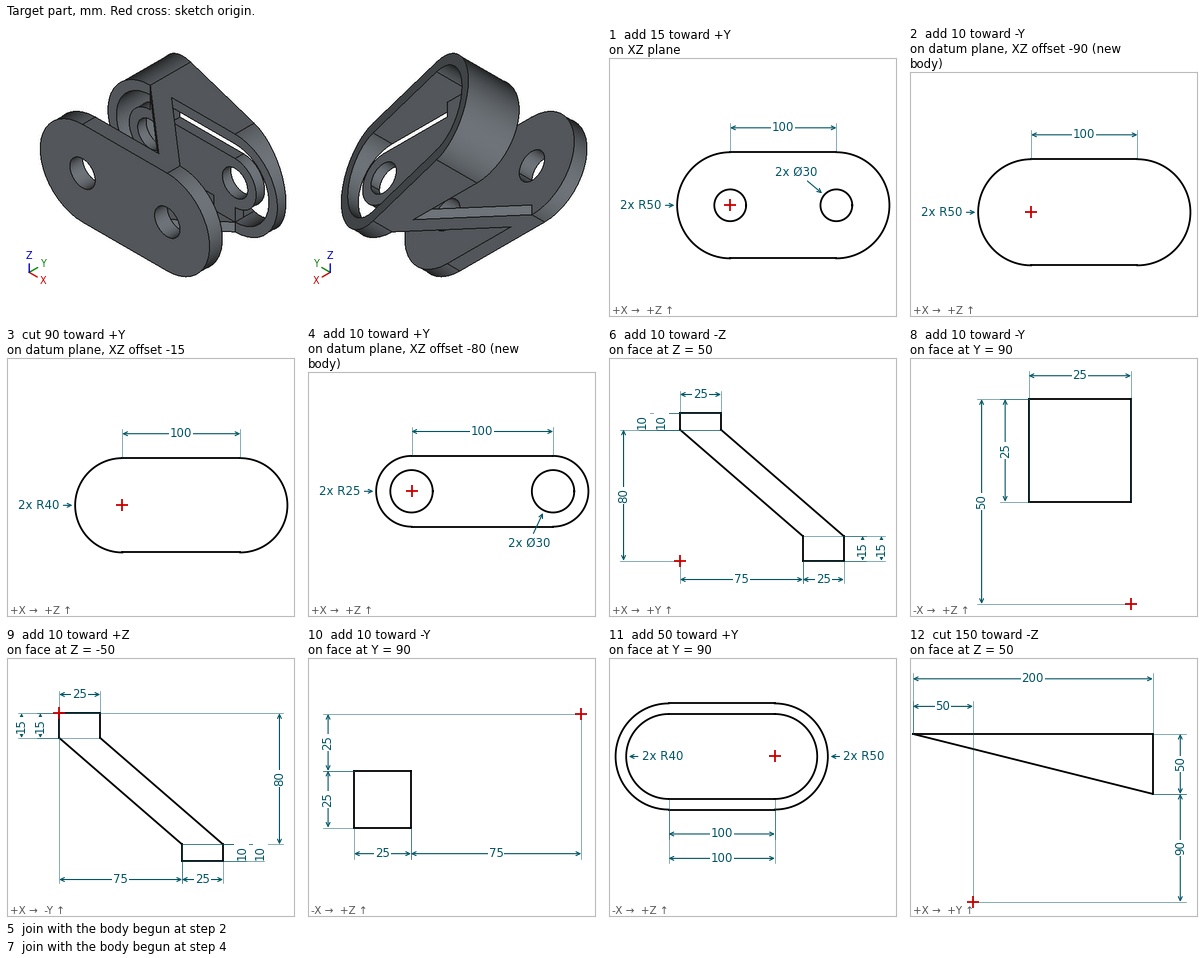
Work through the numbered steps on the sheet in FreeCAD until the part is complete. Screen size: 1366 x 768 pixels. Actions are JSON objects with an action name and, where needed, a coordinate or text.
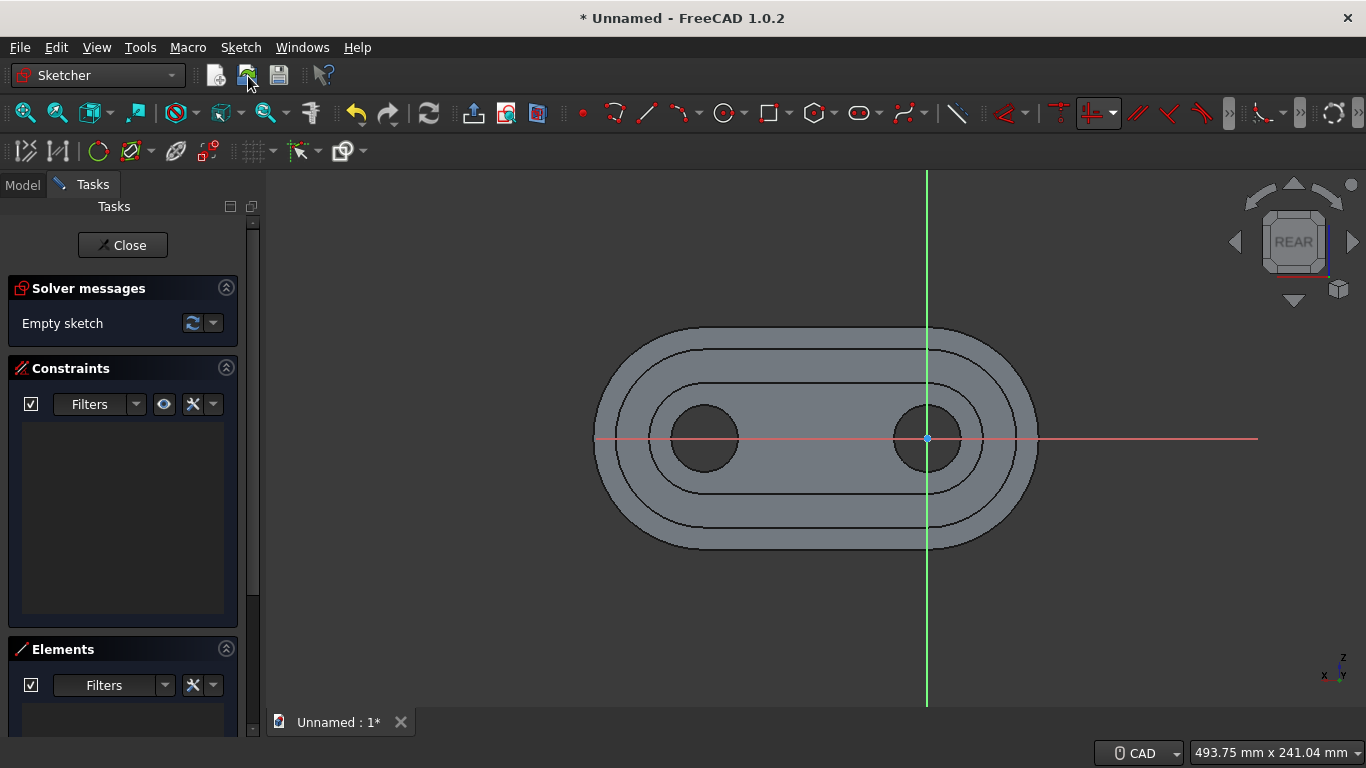
{"action": "scroll", "coordinate": [965, 359], "scroll_direction": "up", "scroll_amount": 6}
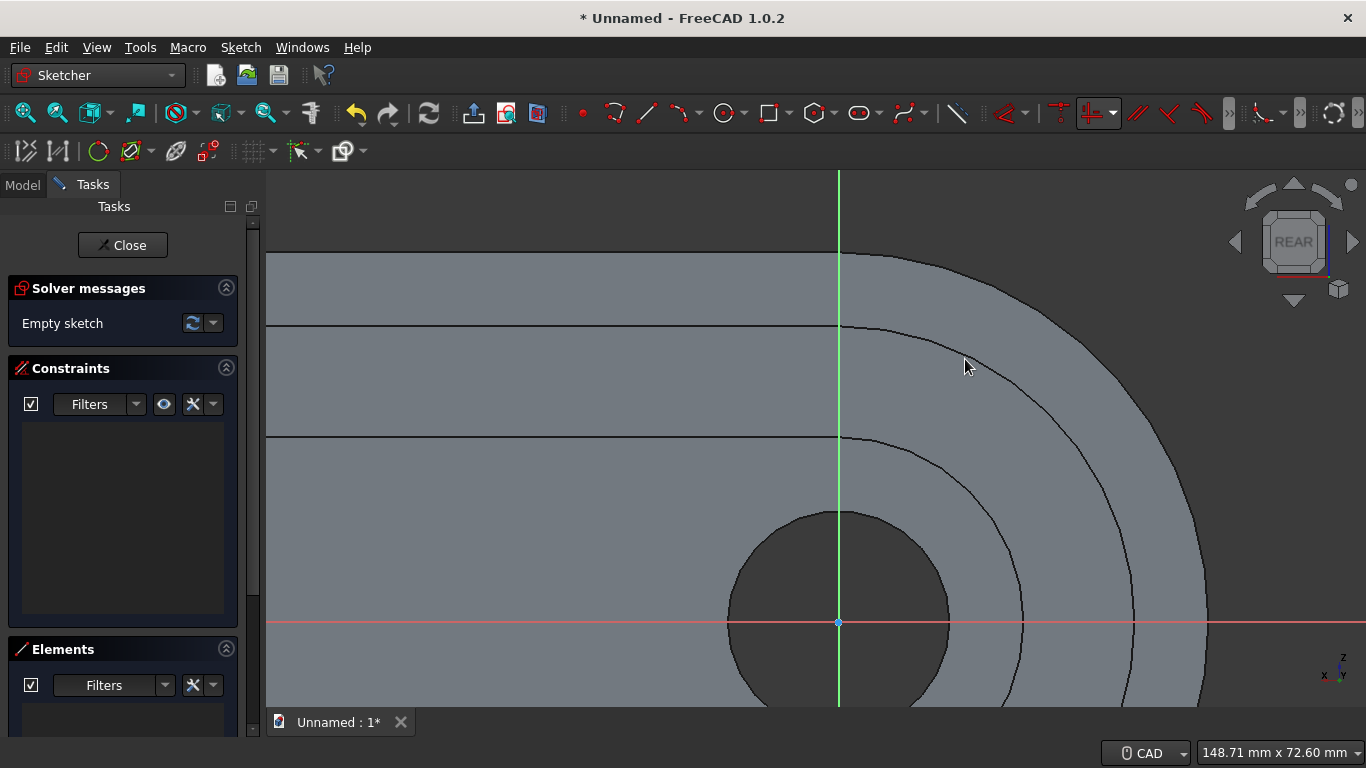
{"action": "left_click", "coordinate": [770, 114]}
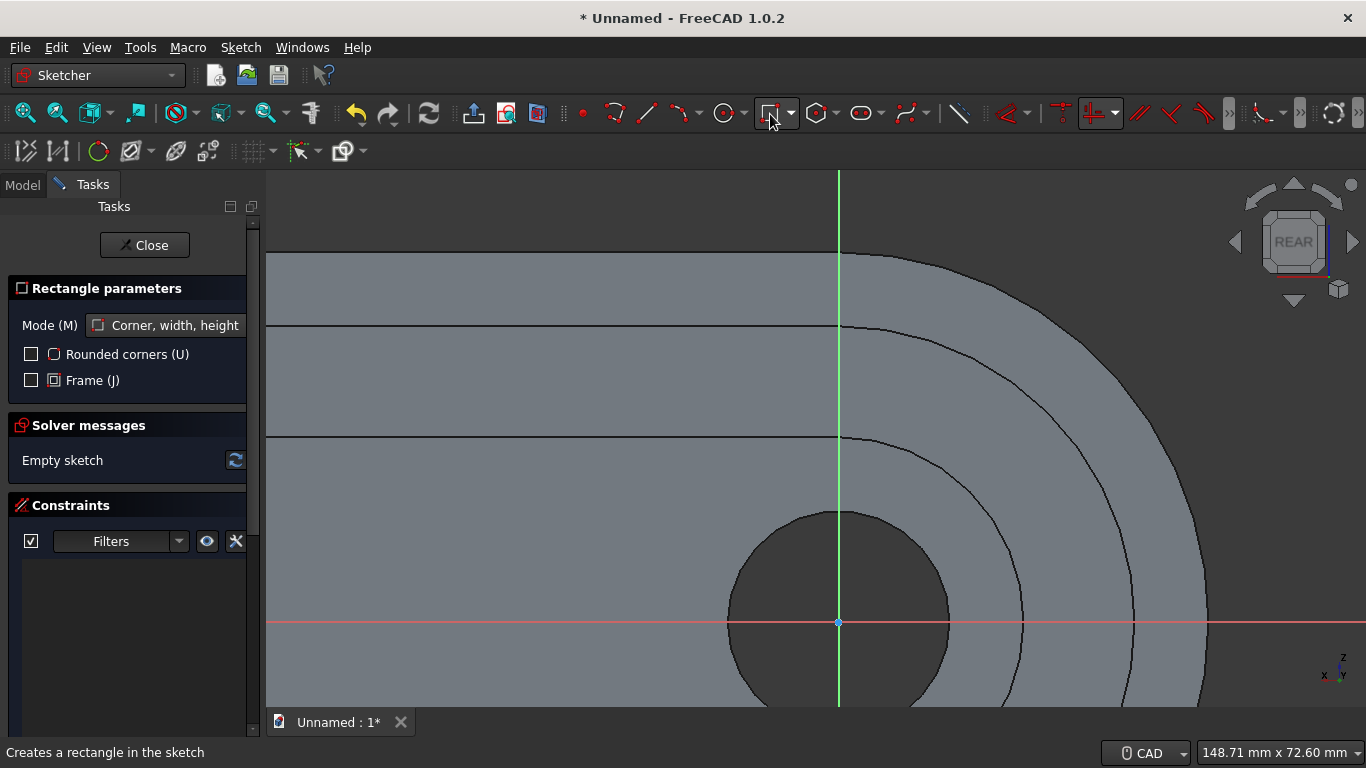
{"action": "left_click", "coordinate": [654, 252]}
{"action": "left_click", "coordinate": [839, 437]}
{"action": "key", "text": "Escape"}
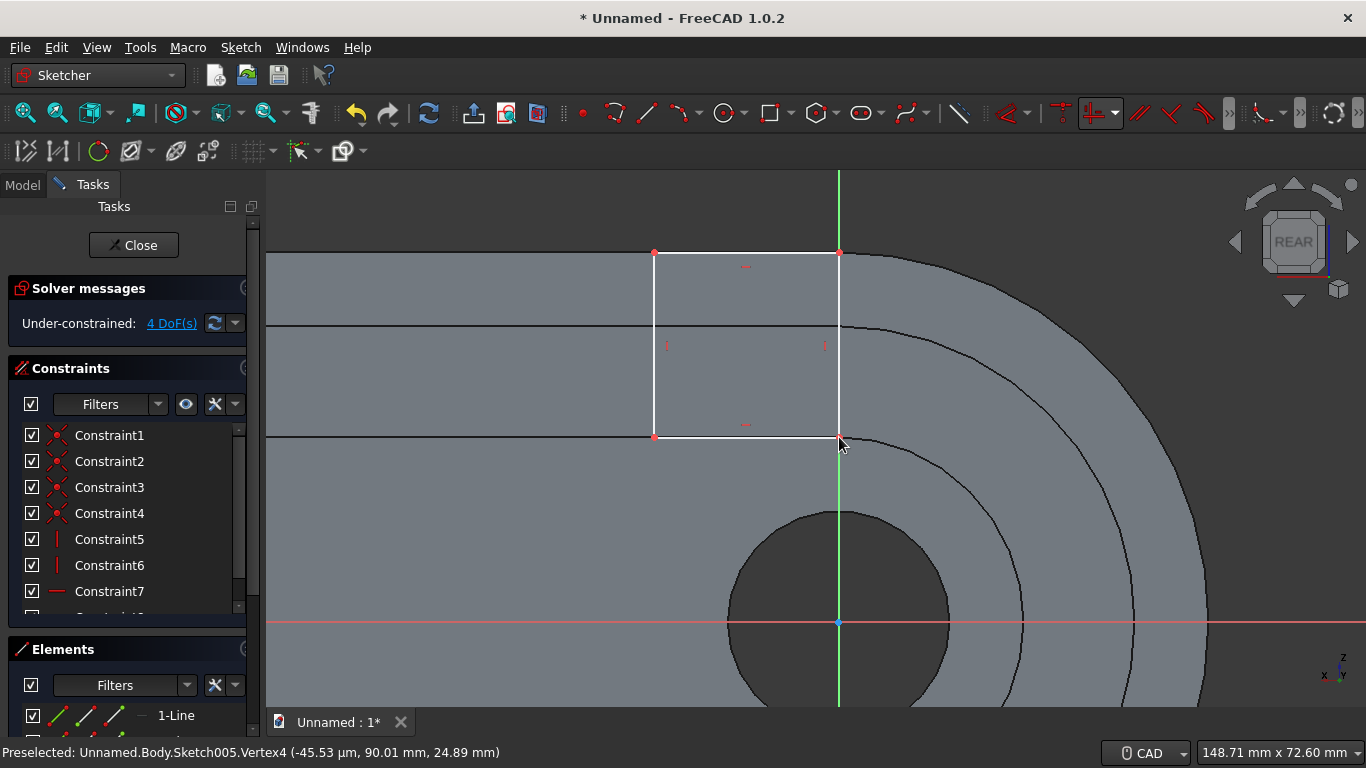
{"action": "left_click", "coordinate": [839, 438]}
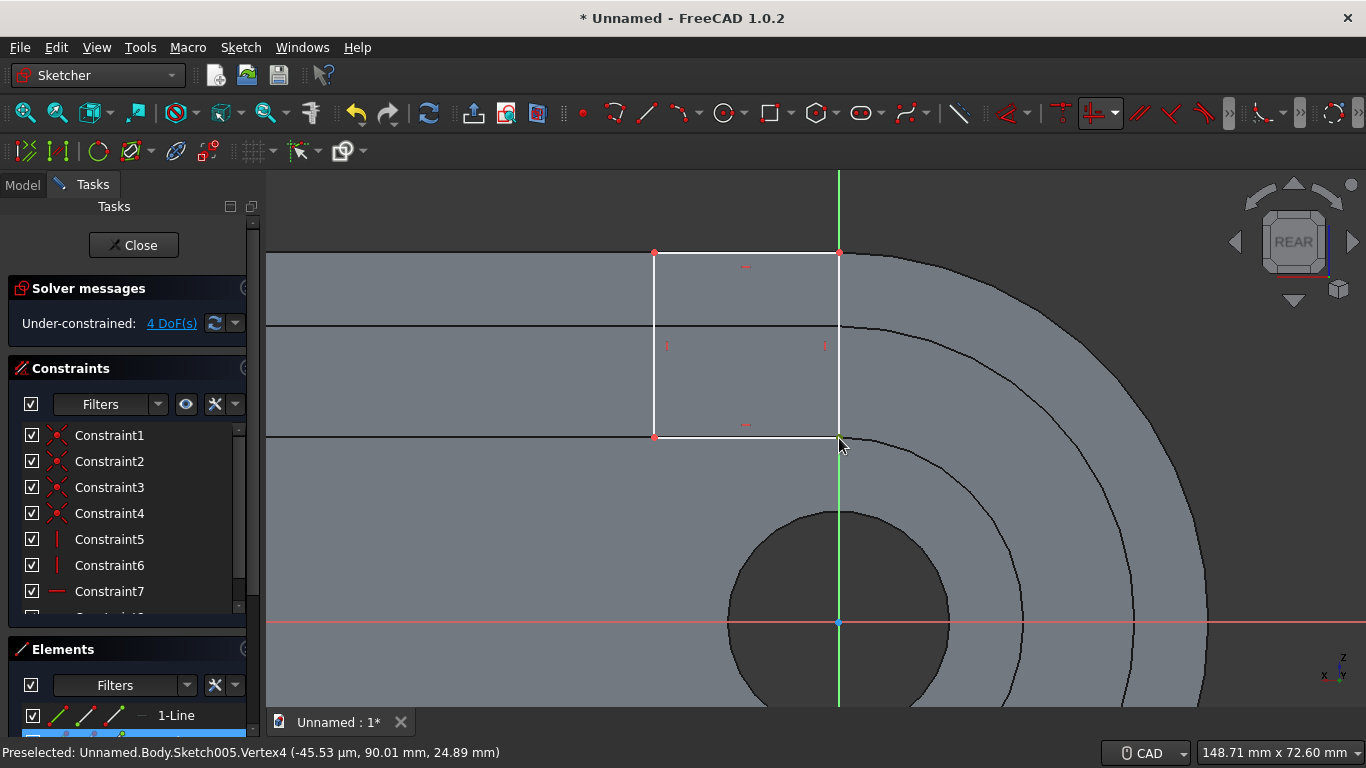
{"action": "left_click", "coordinate": [839, 576]}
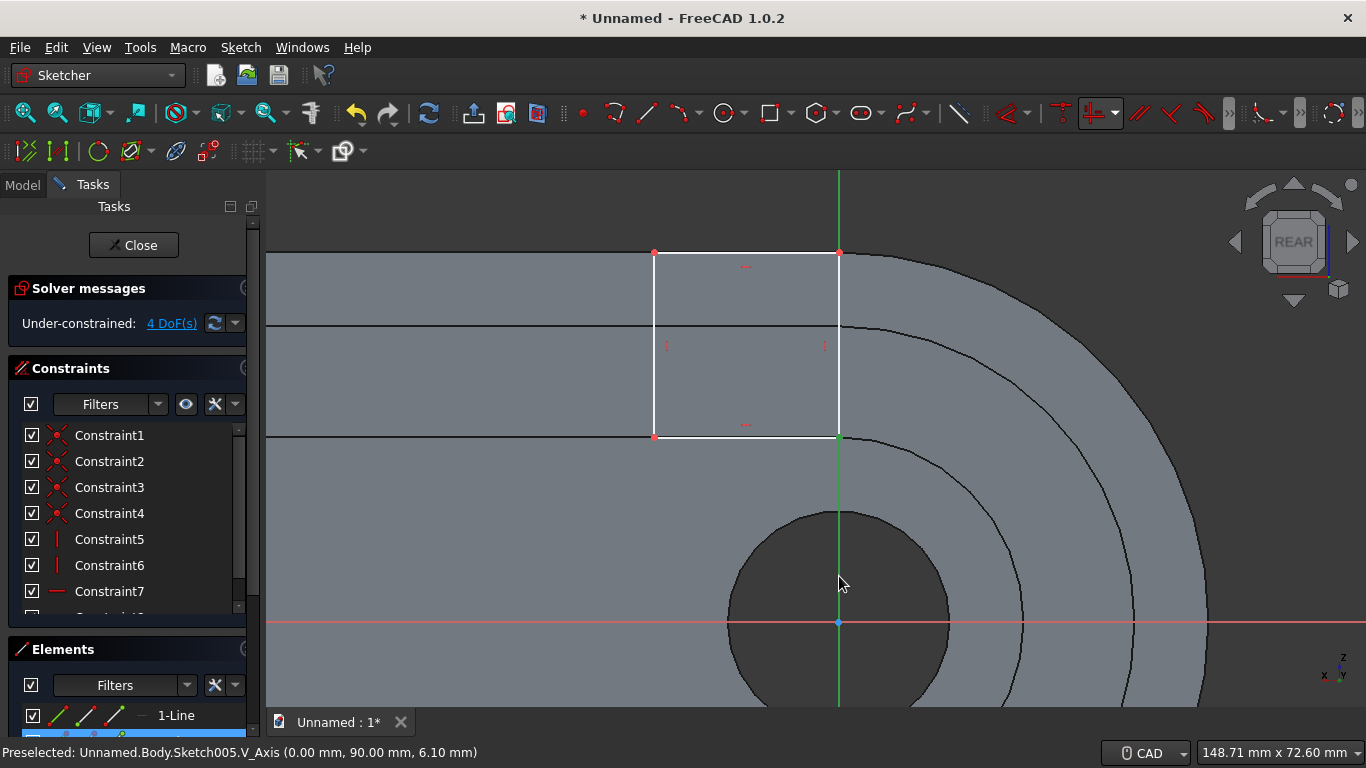
{"action": "left_click", "coordinate": [1062, 114]}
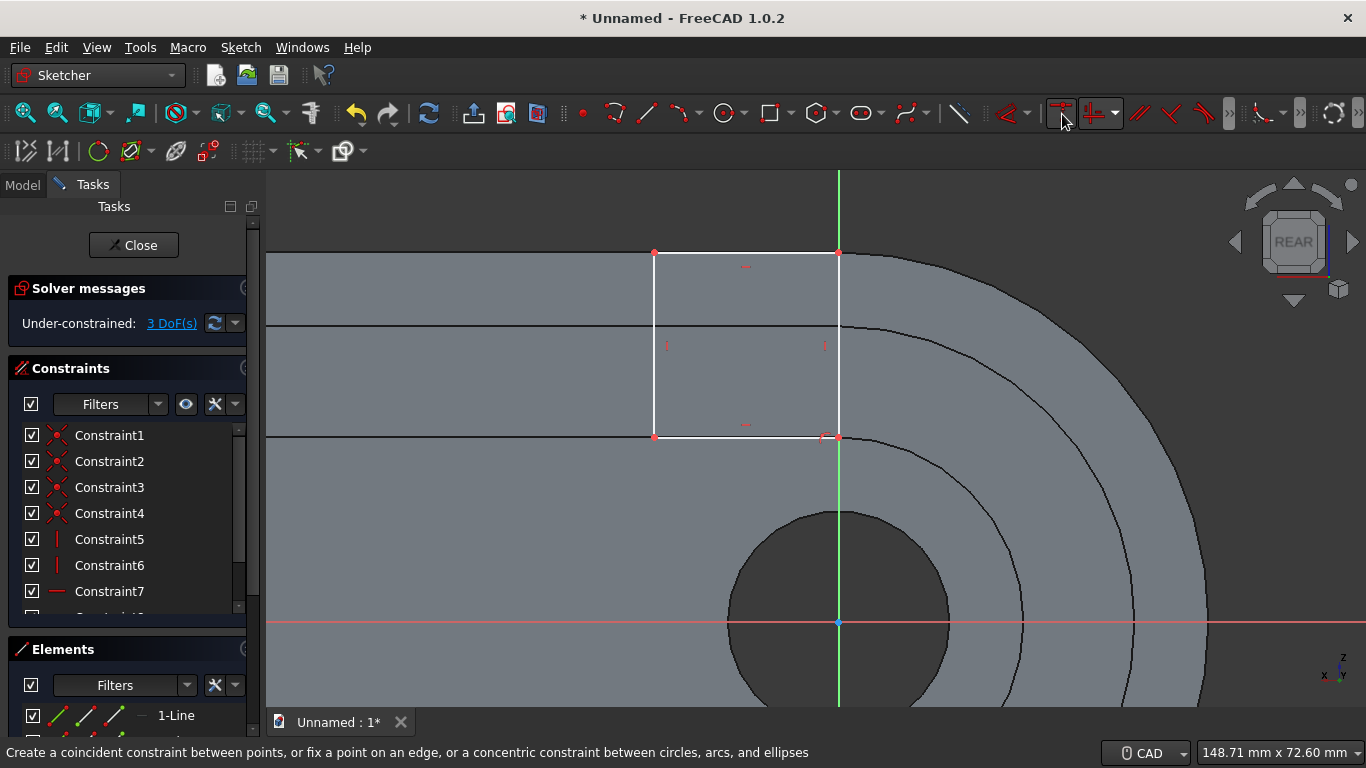
{"action": "left_click", "coordinate": [1006, 114]}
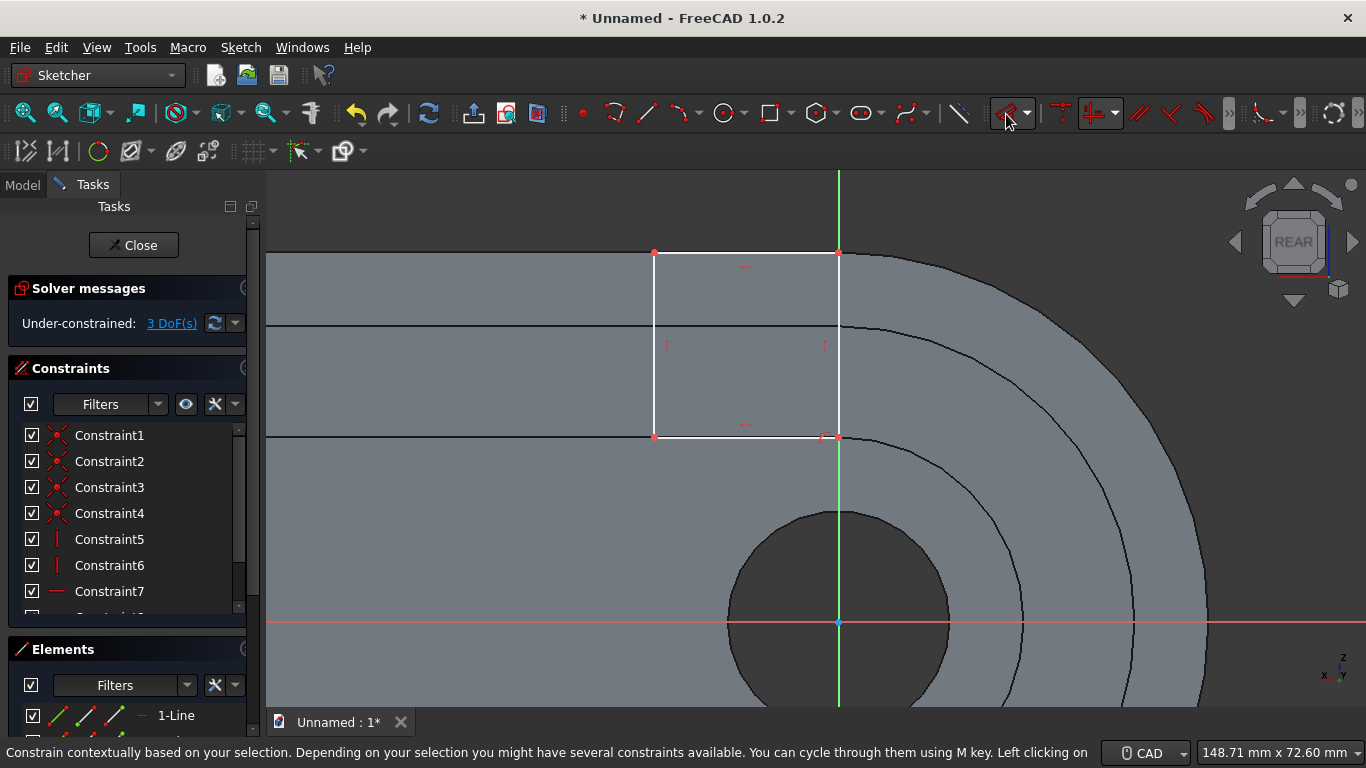
{"action": "left_click", "coordinate": [654, 308]}
{"action": "left_click", "coordinate": [620, 346]}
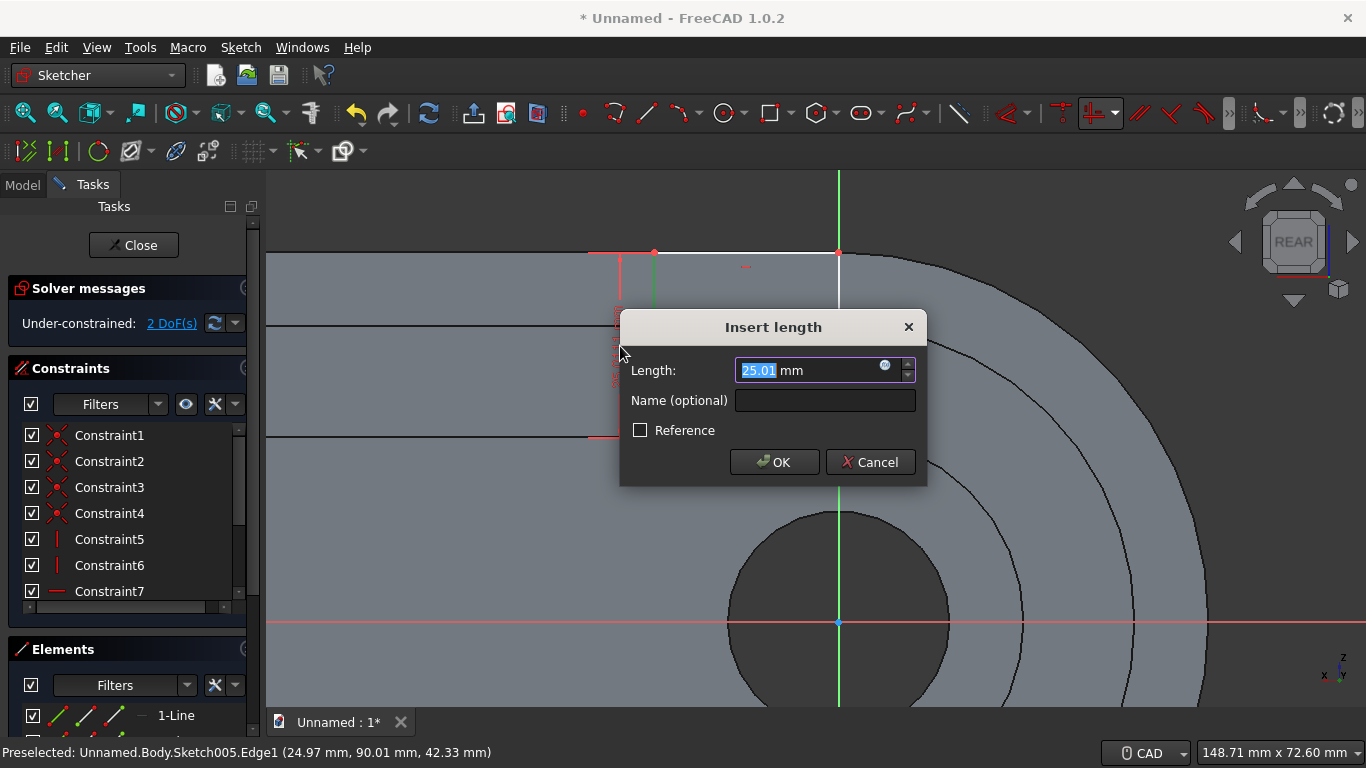
{"action": "type", "text": "25"}
{"action": "key", "text": "Return"}